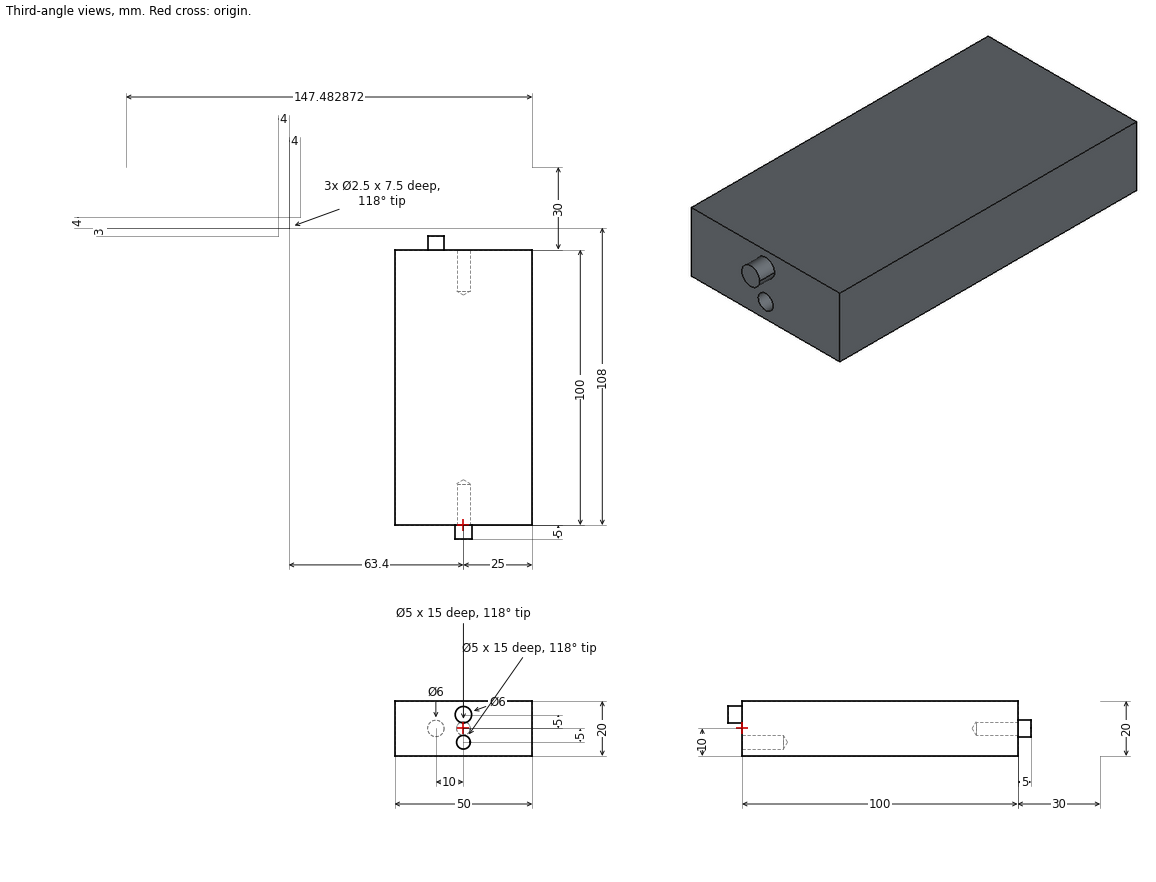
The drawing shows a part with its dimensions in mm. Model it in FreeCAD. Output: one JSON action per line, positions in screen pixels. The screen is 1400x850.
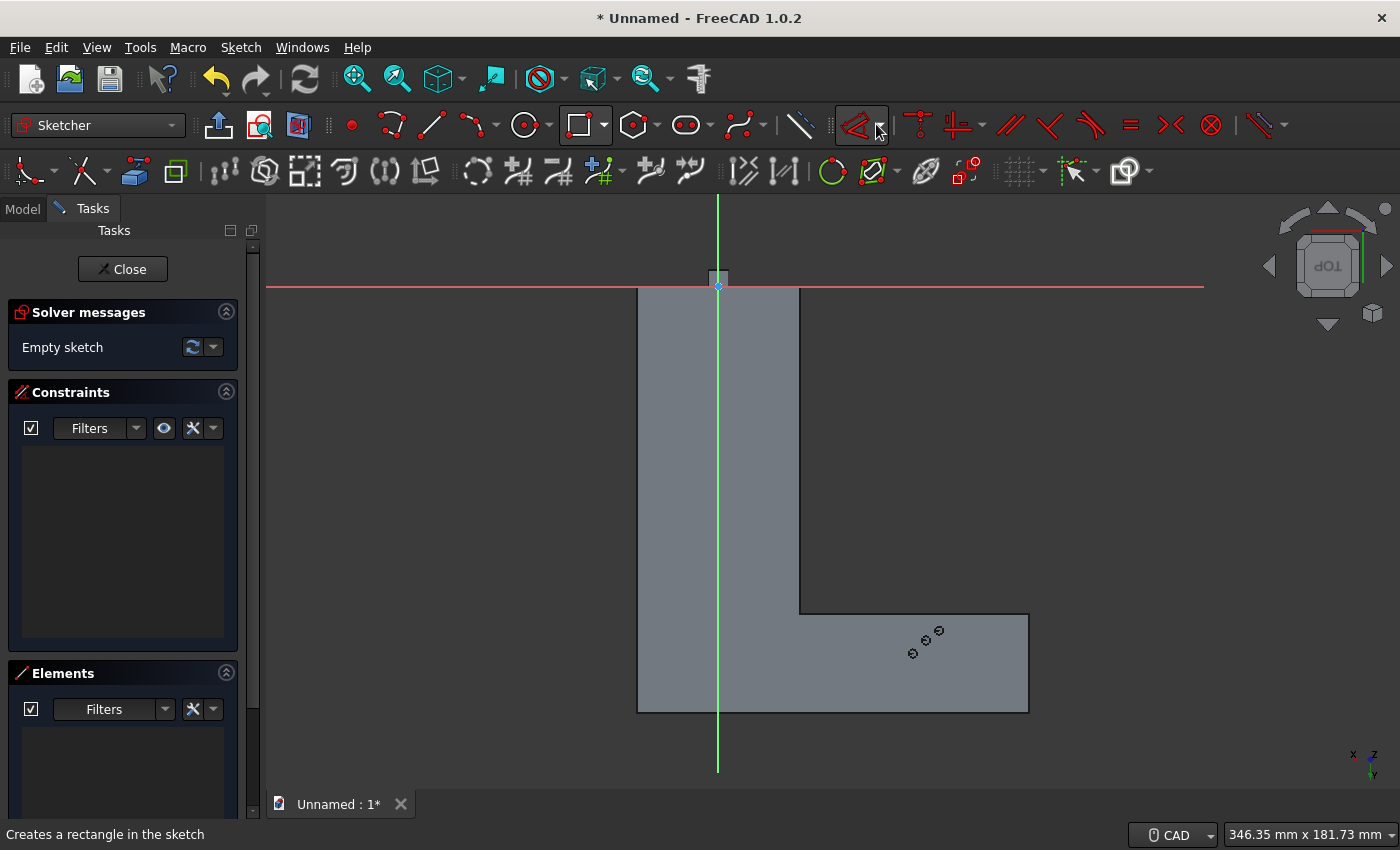
{"action": "left_click", "coordinate": [580, 126]}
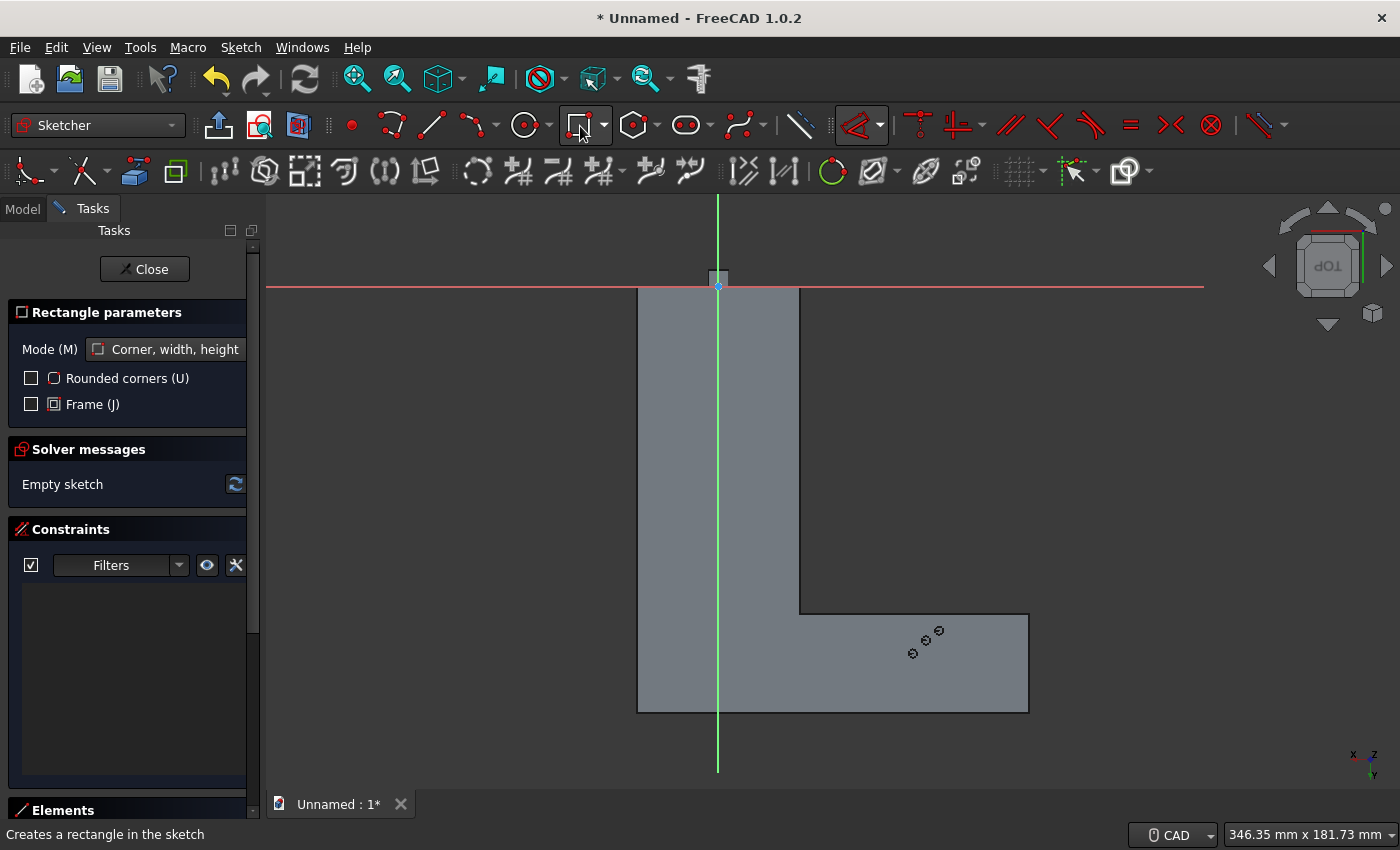
{"action": "left_click", "coordinate": [637, 614]}
{"action": "left_click", "coordinate": [1119, 713]}
{"action": "key", "text": "Escape"}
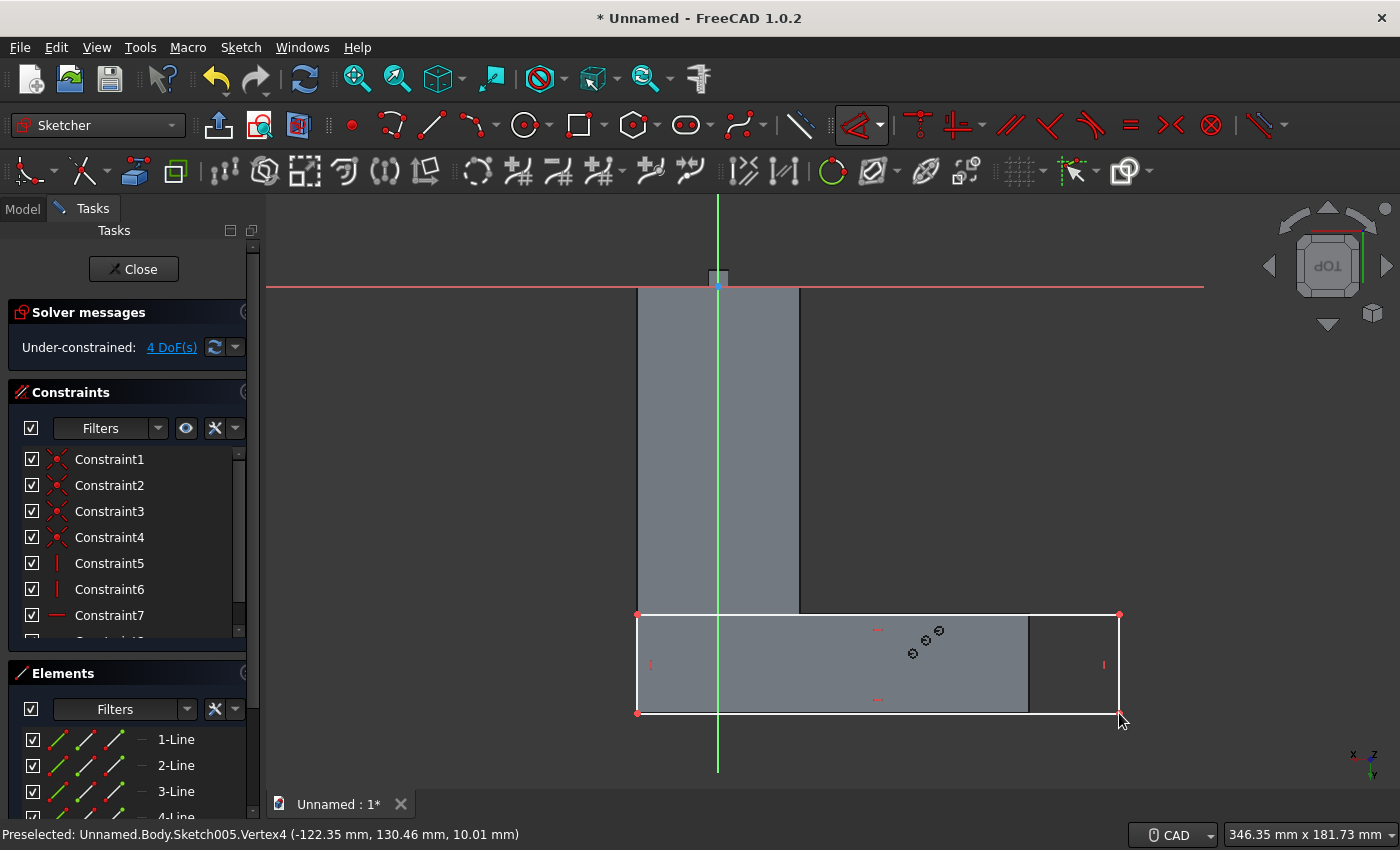
{"action": "left_click", "coordinate": [637, 645]}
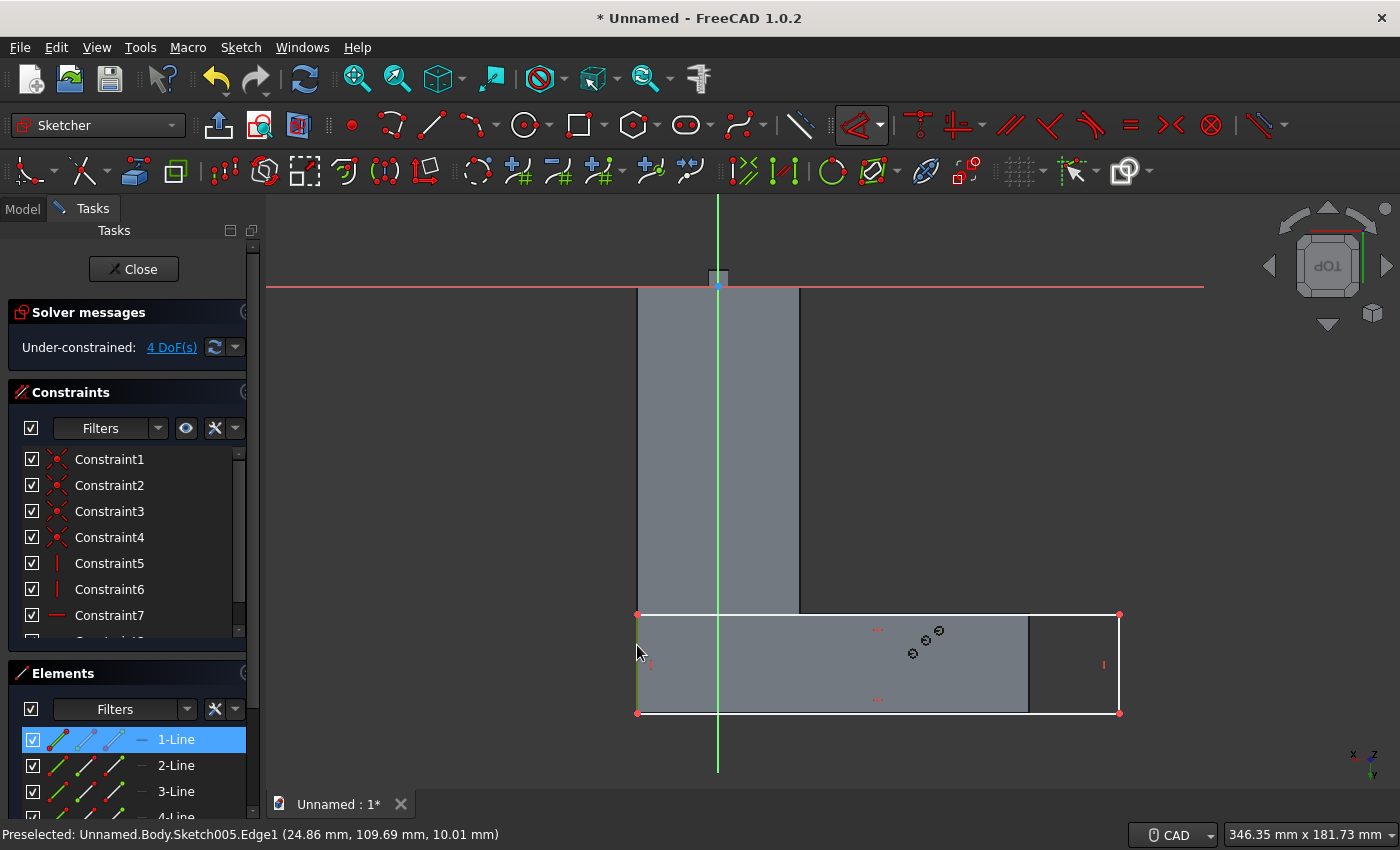
{"action": "key", "text": "i"}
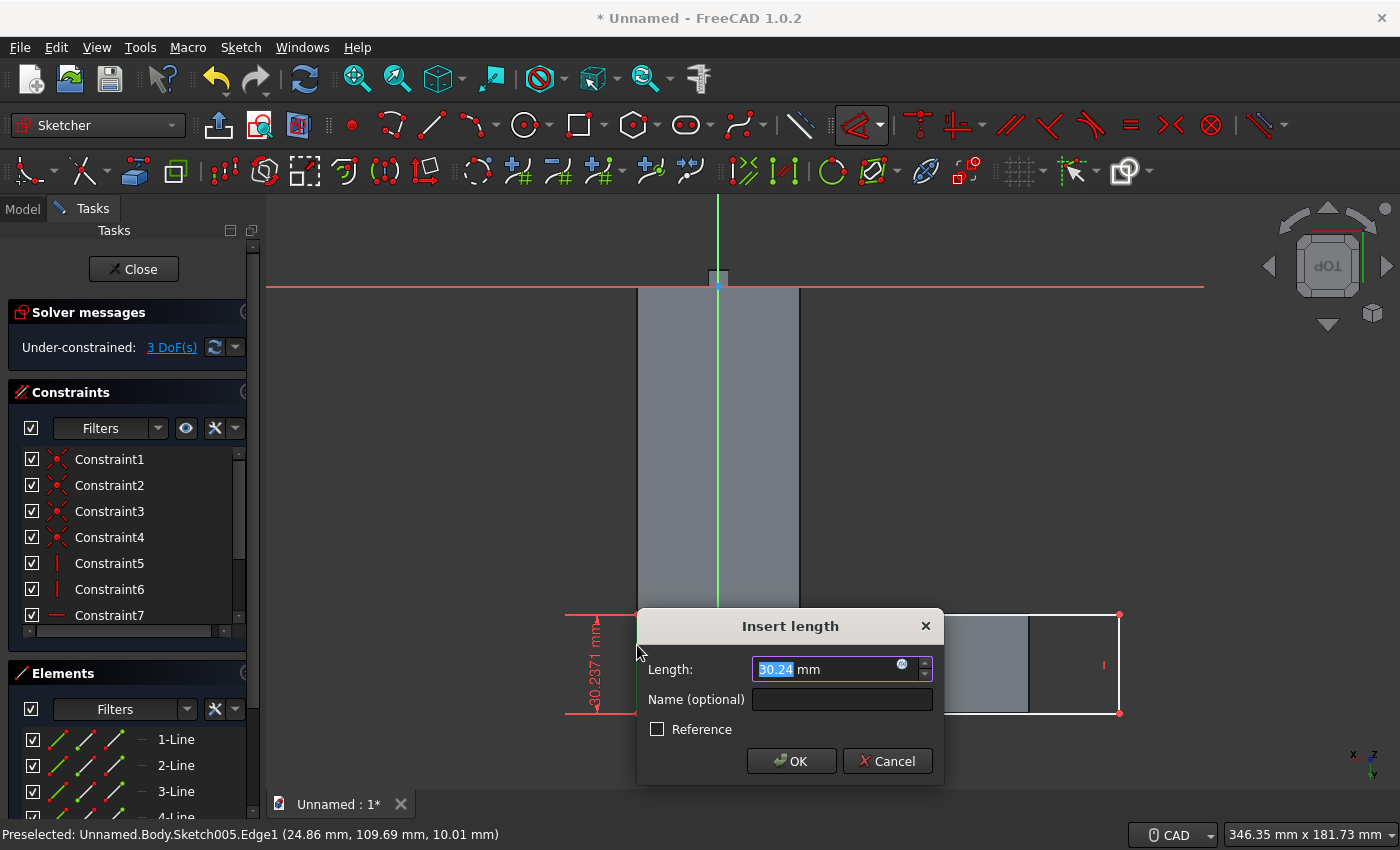
{"action": "type", "text": "30"}
{"action": "key", "text": "Return"}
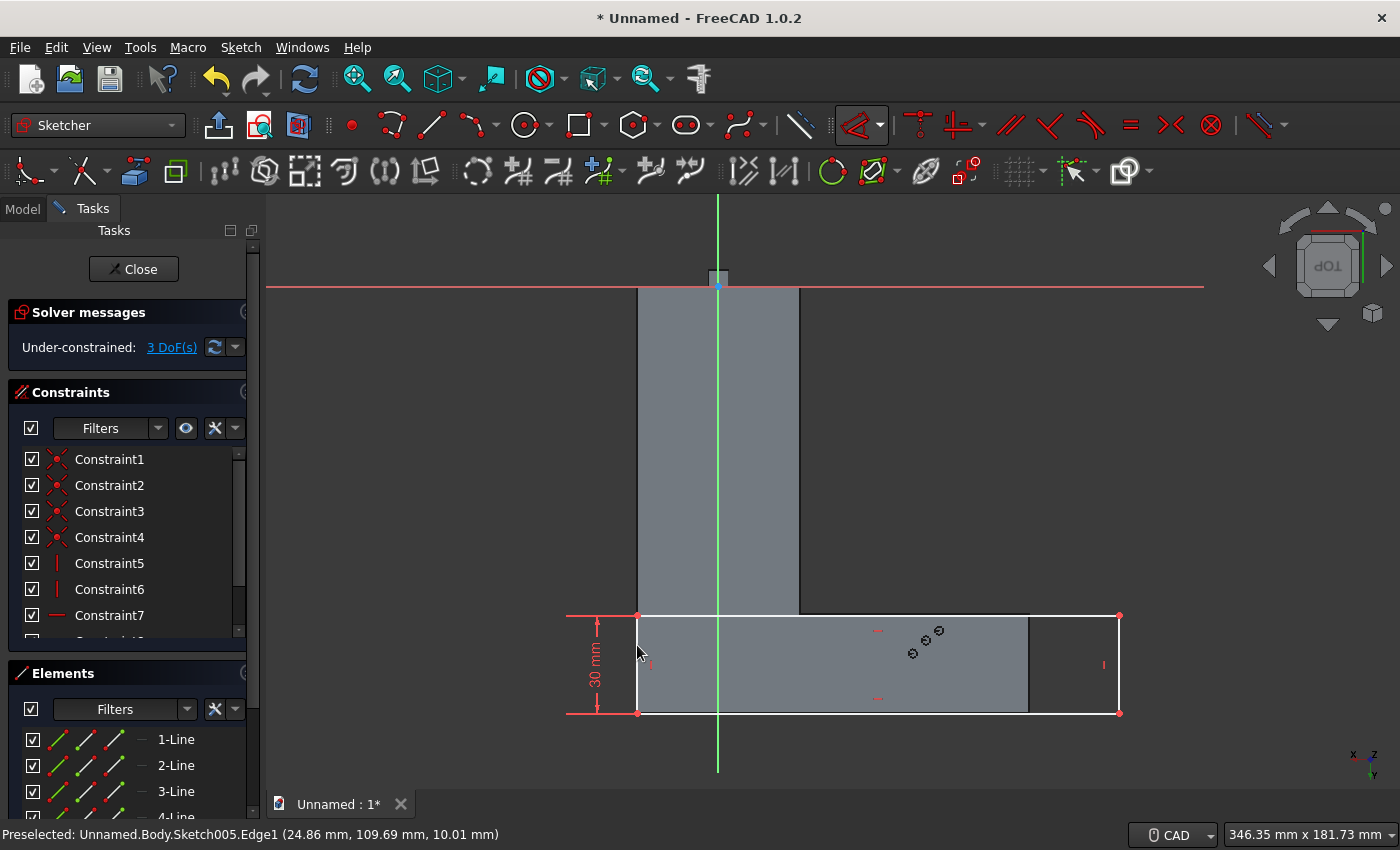
{"action": "left_click", "coordinate": [637, 616]}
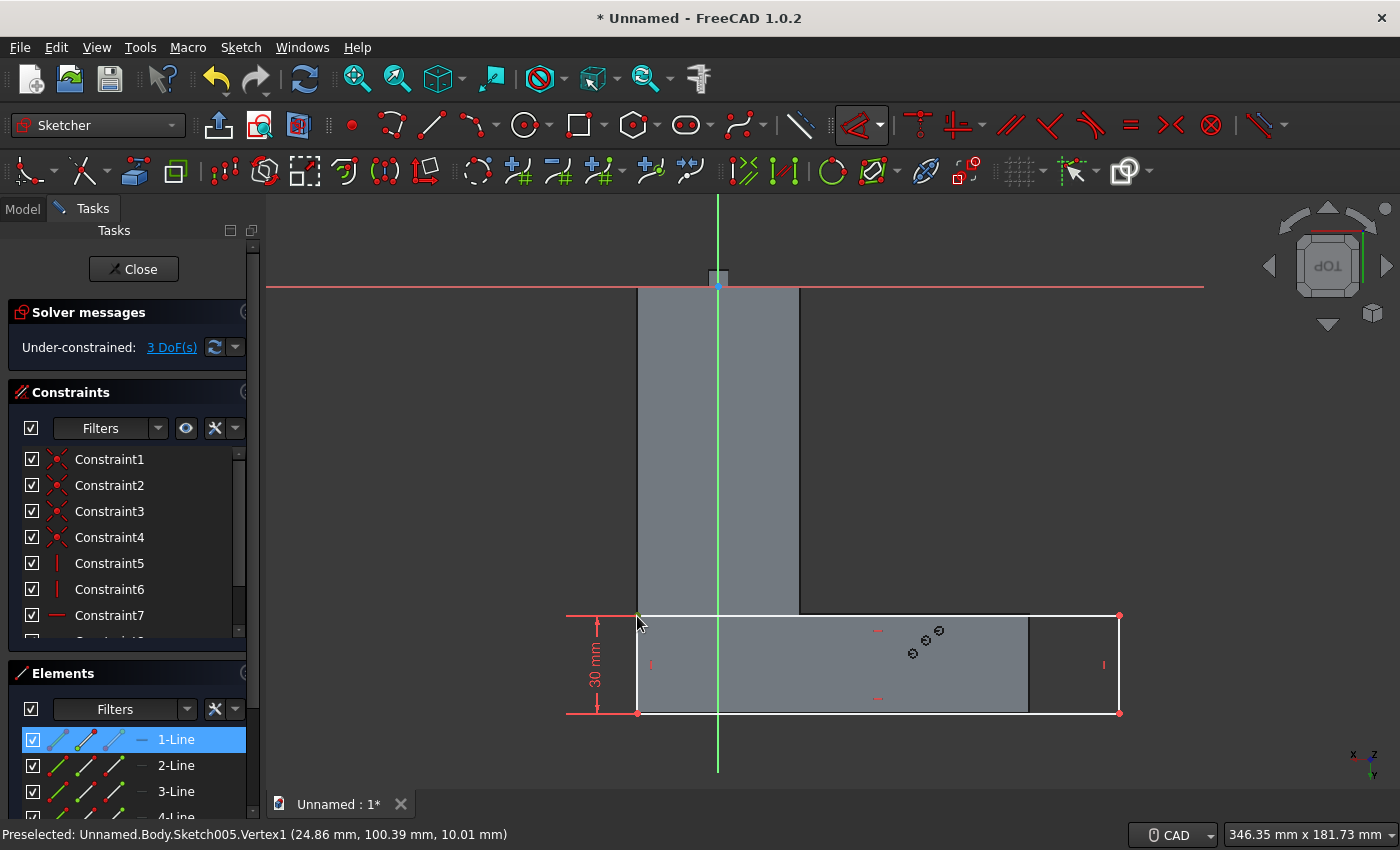
{"action": "left_click", "coordinate": [882, 126]}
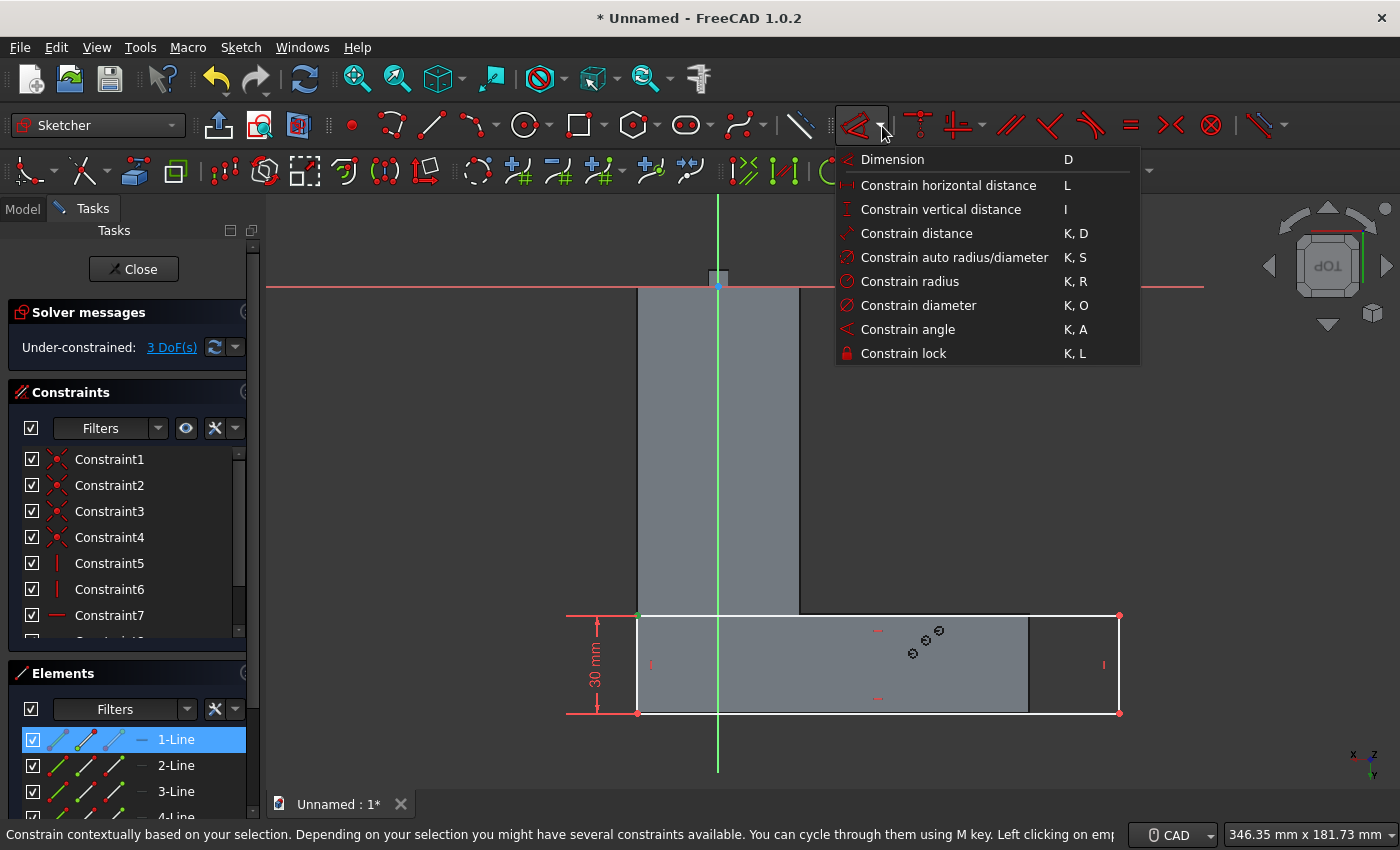
{"action": "left_click", "coordinate": [988, 185]}